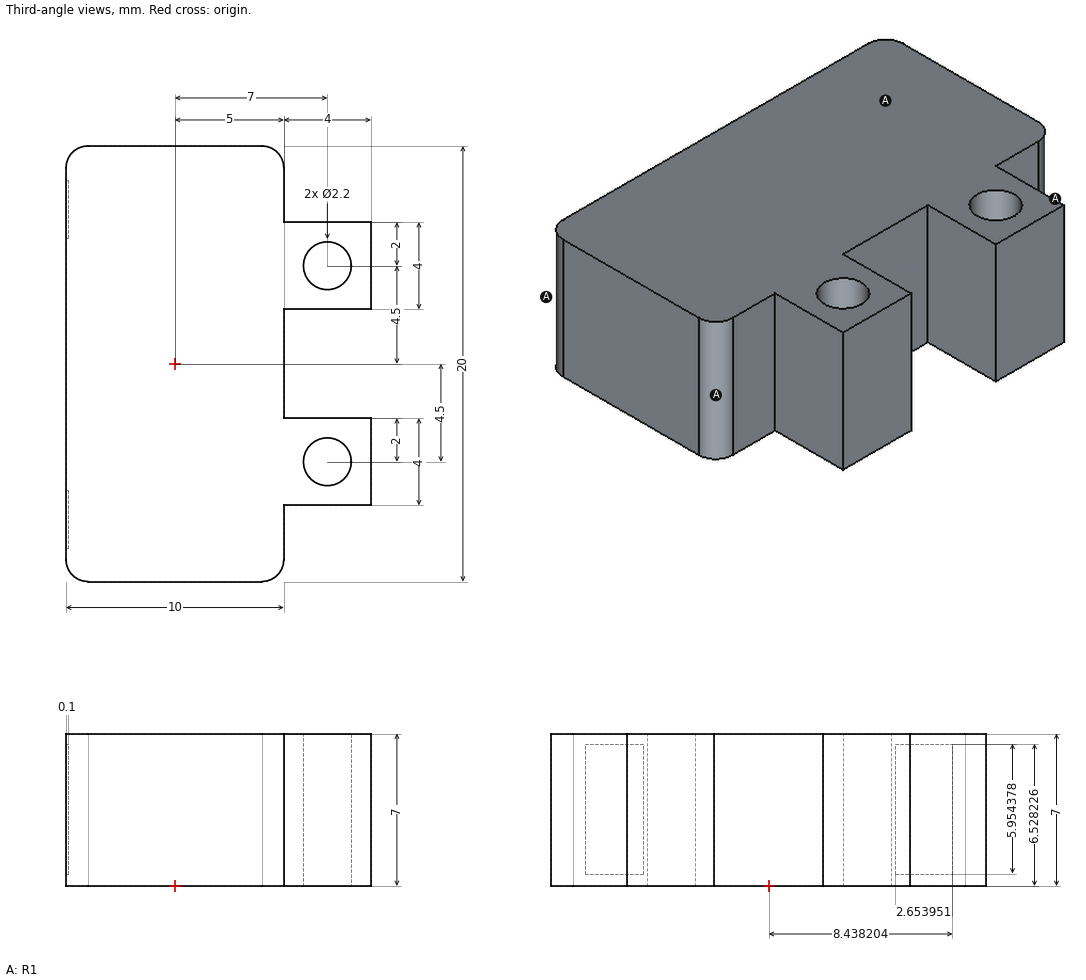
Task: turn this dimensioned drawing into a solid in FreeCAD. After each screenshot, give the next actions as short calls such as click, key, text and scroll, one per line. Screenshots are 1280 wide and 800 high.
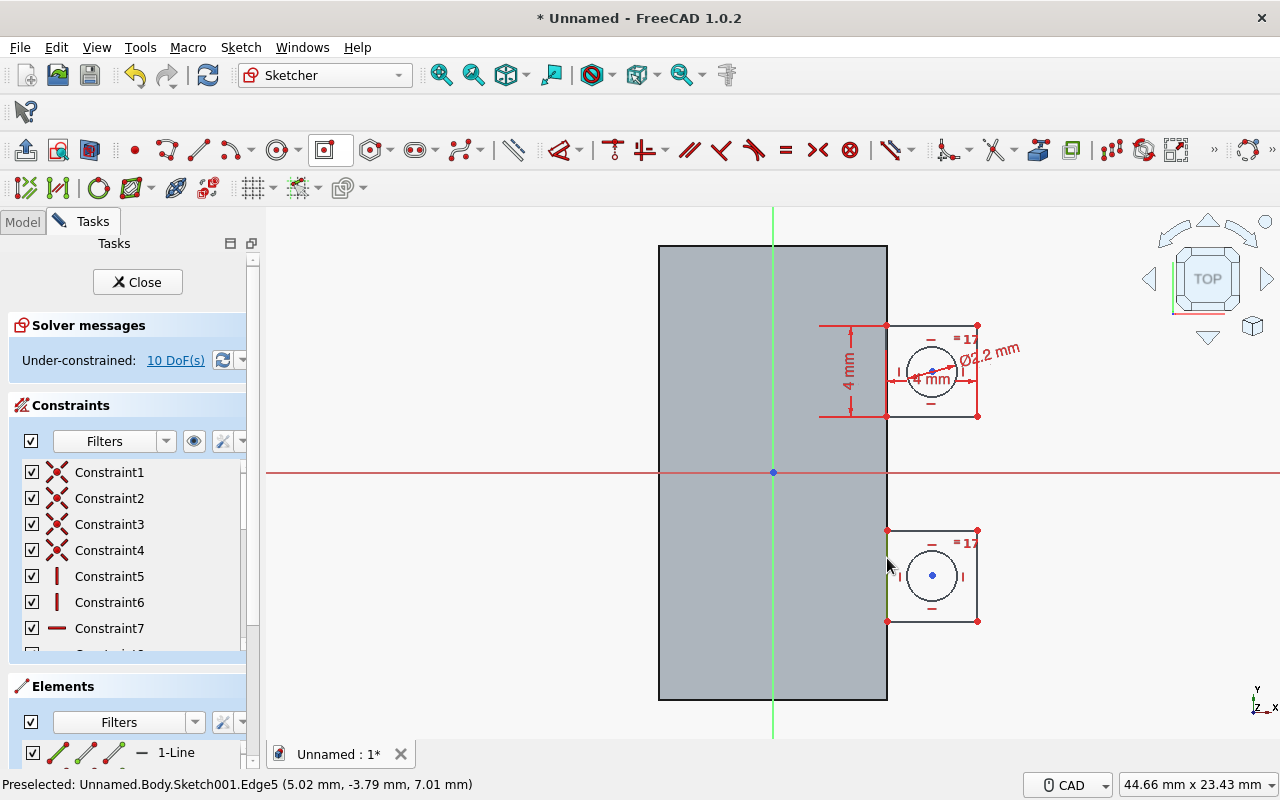
click(582, 150)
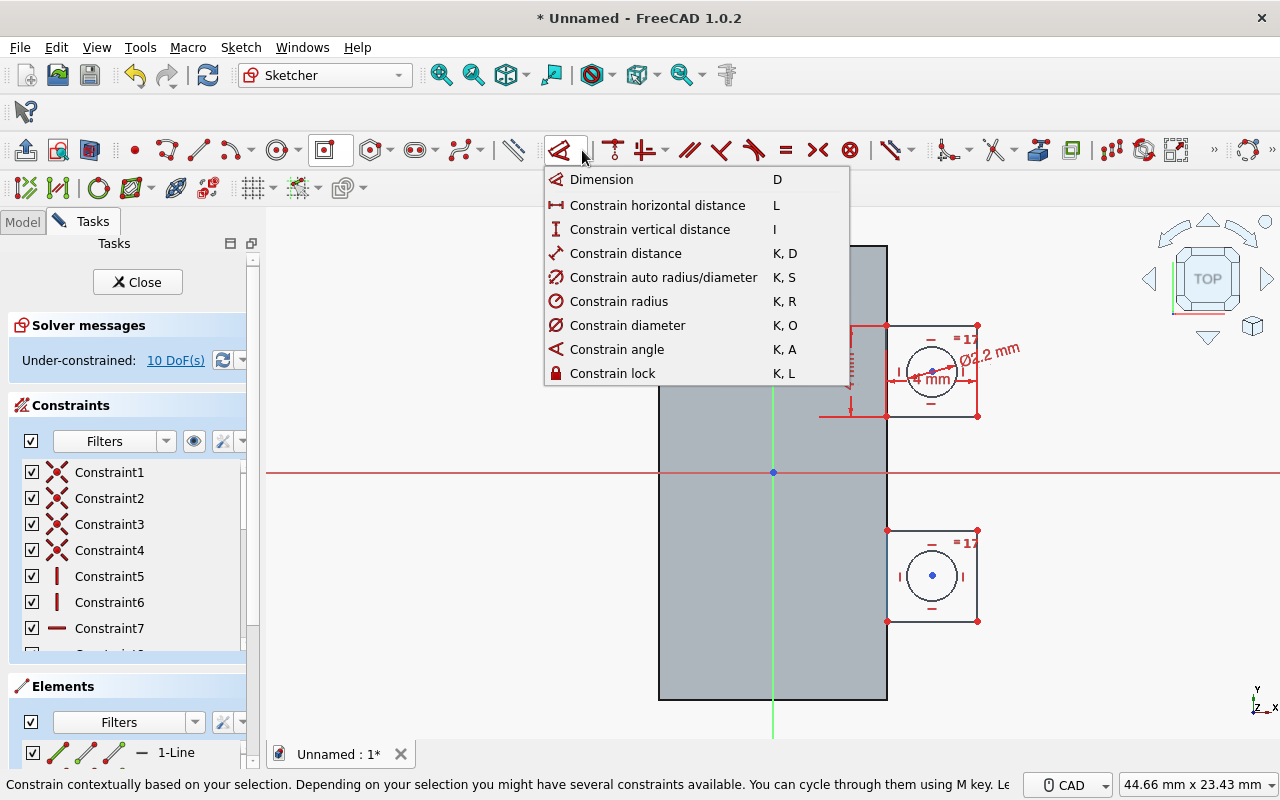
click(697, 229)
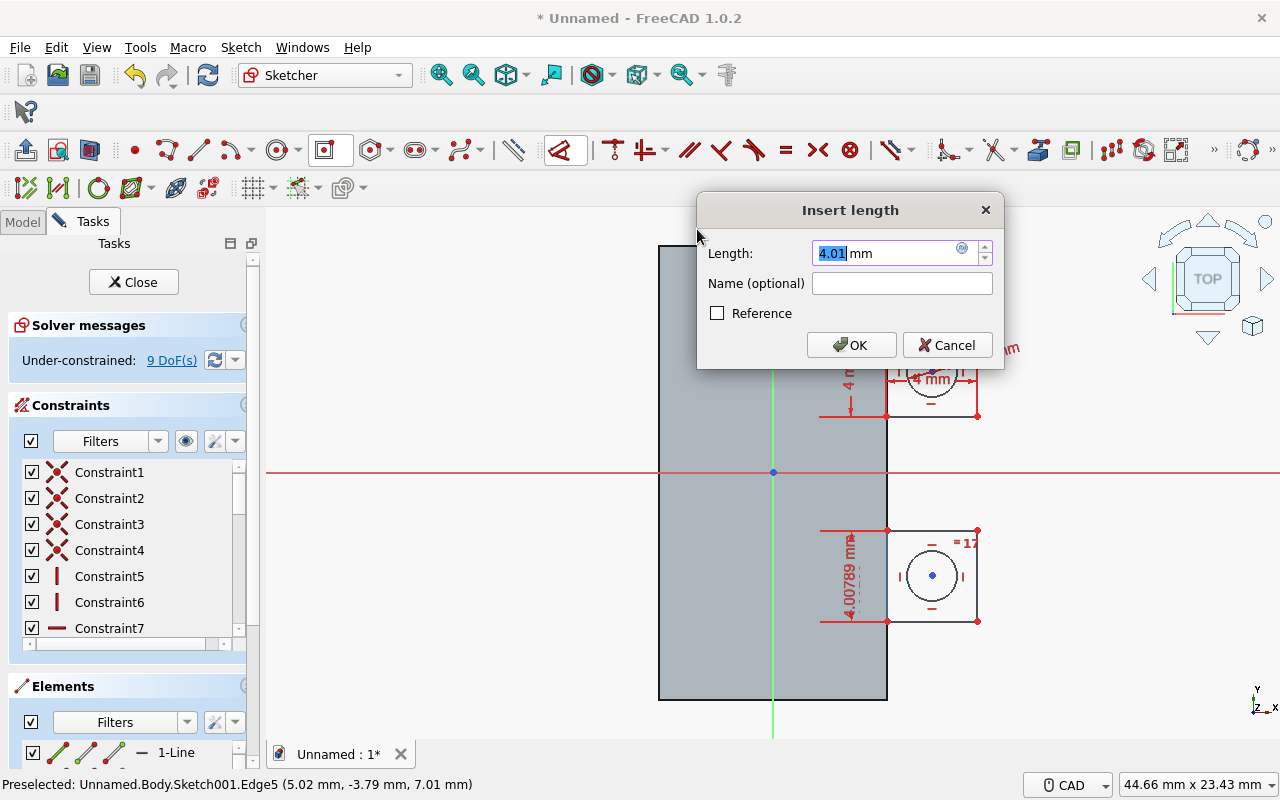
text(4)
key(Return)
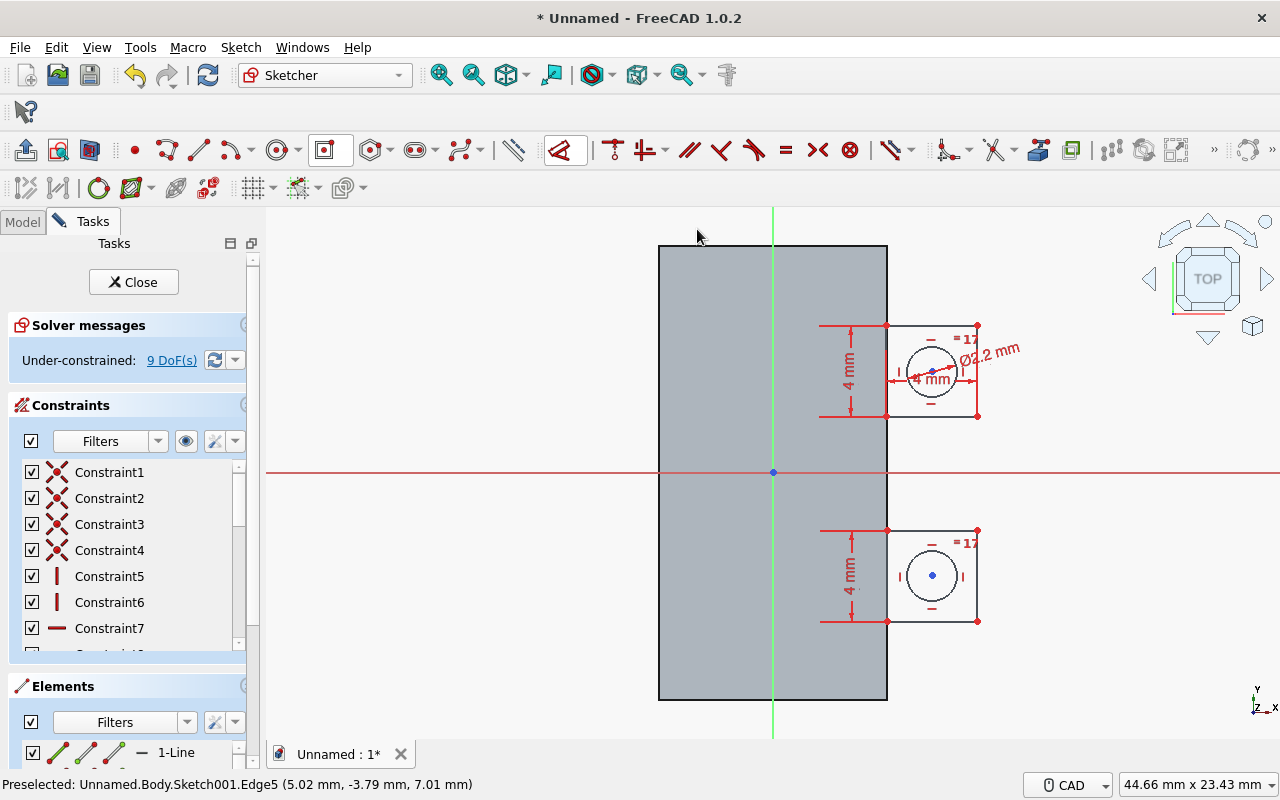
click(914, 622)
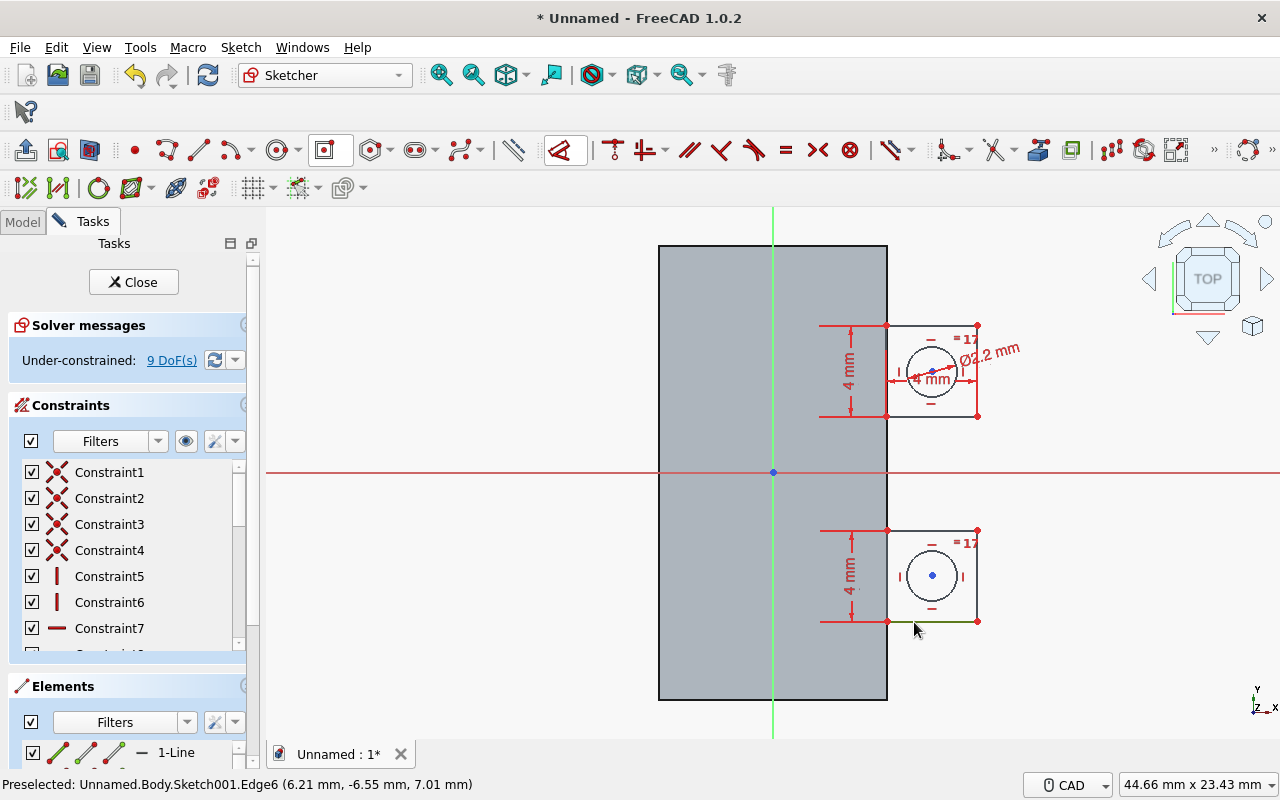
key(l)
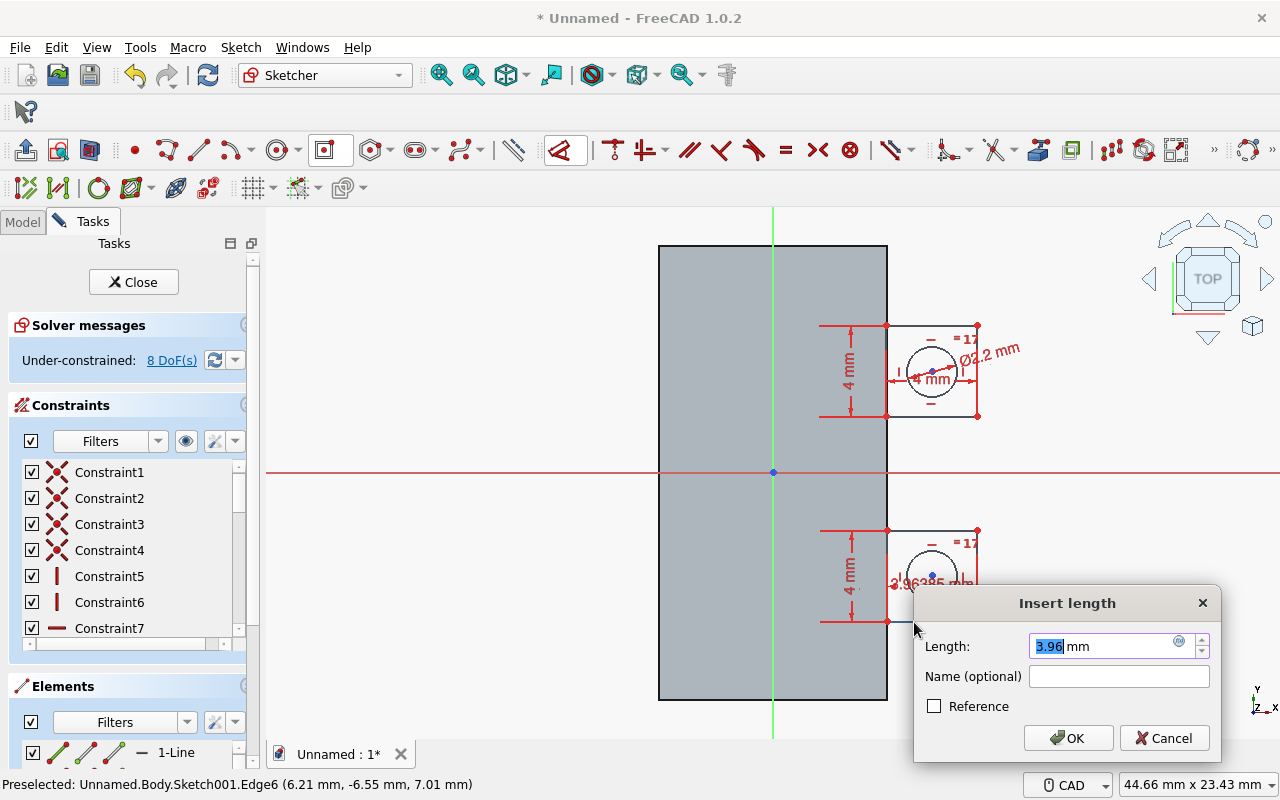
text(4)
key(Return)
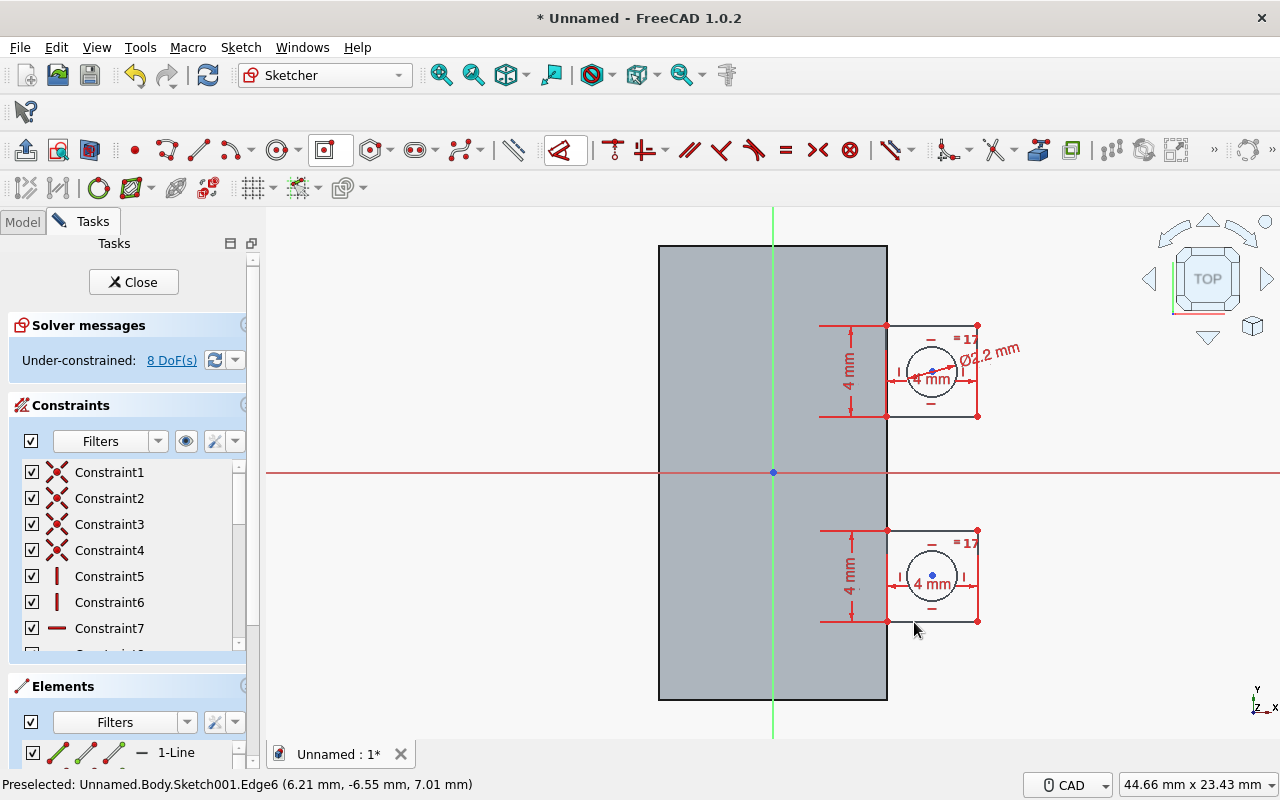
click(932, 372)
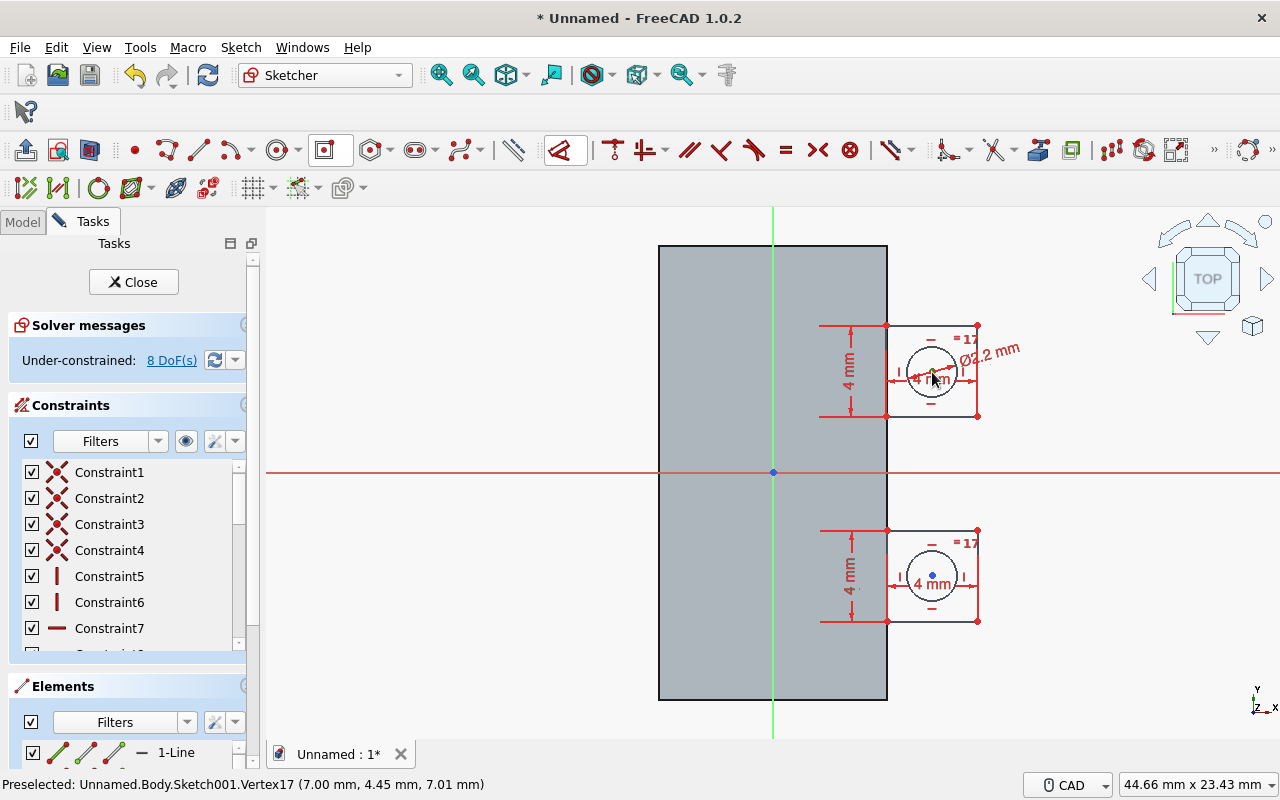
click(582, 150)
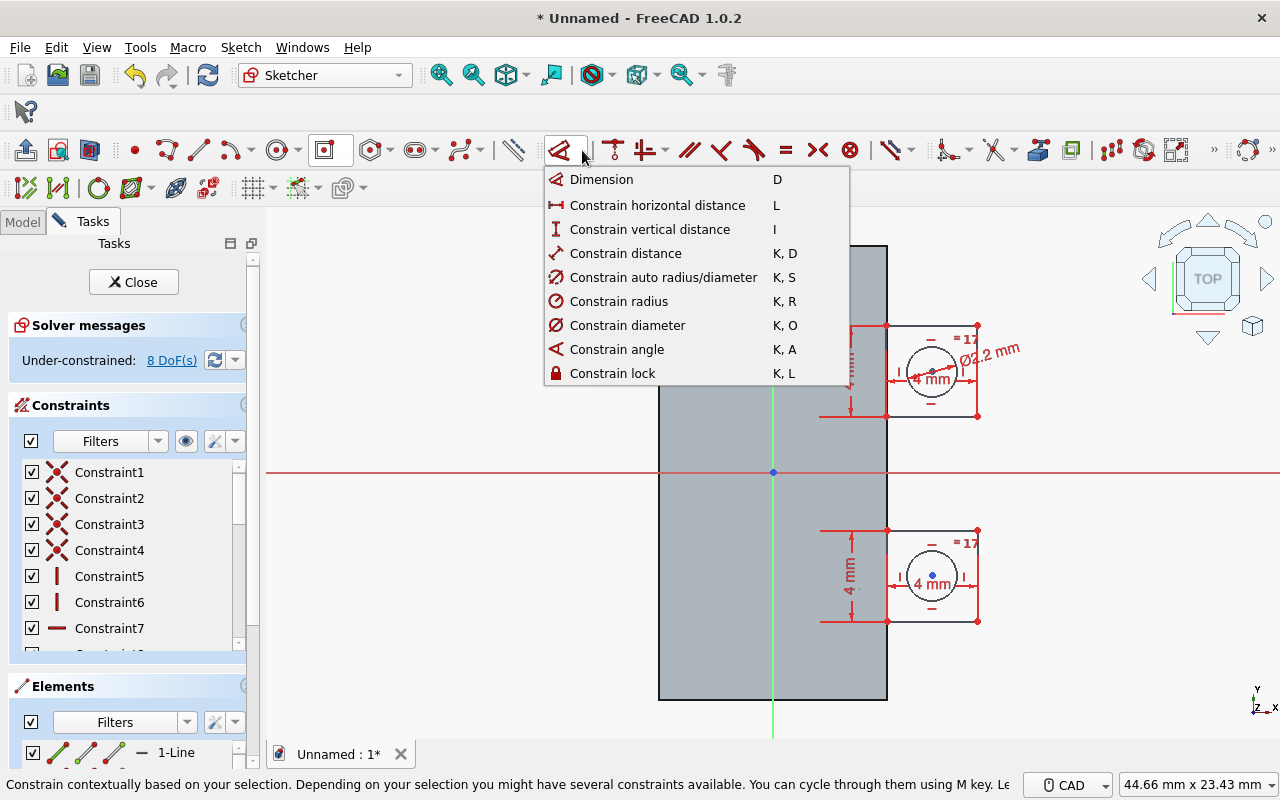
click(697, 205)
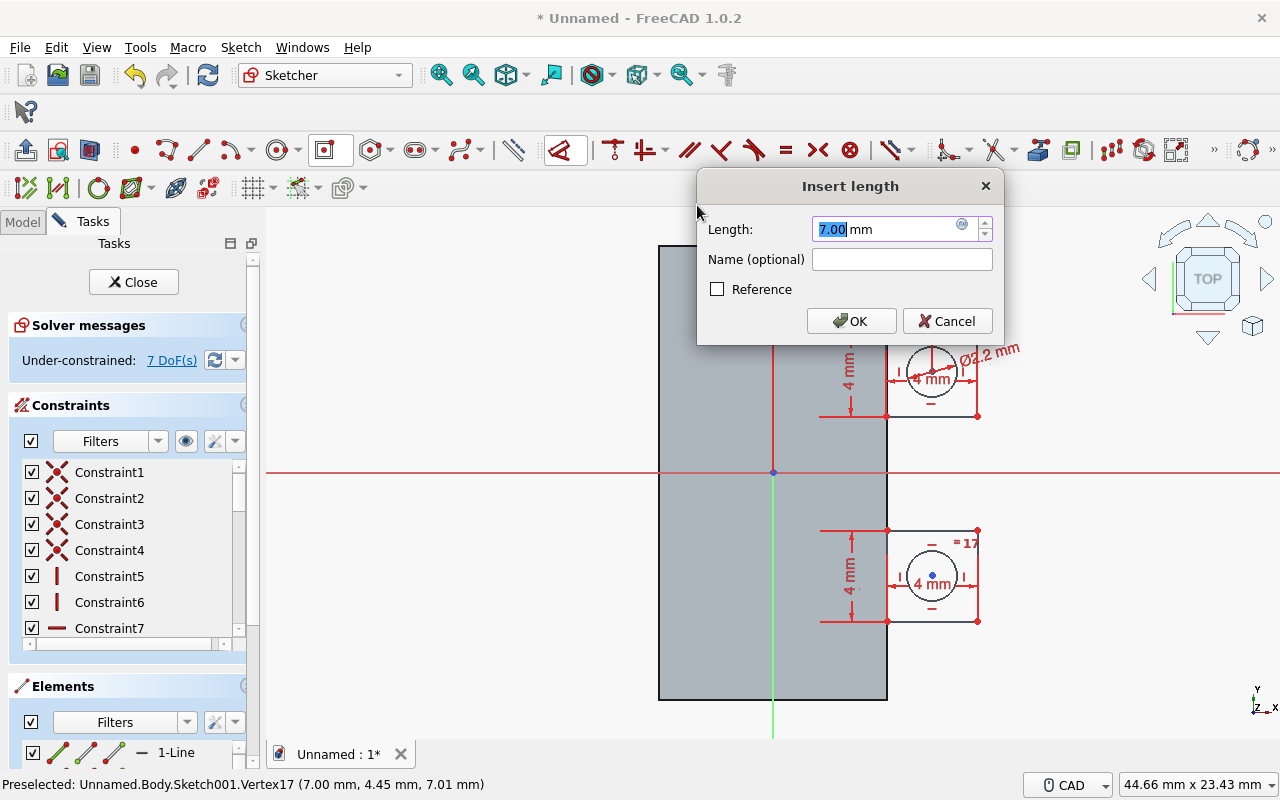
text(7)
key(Return)